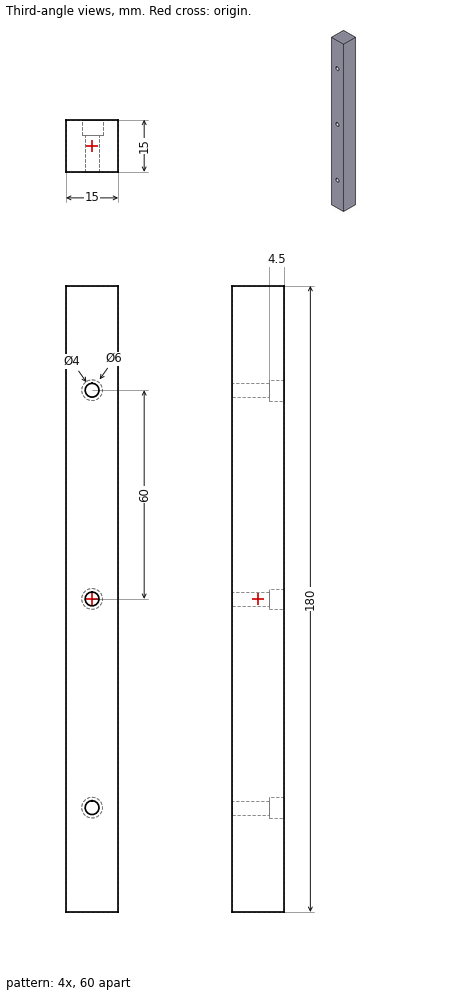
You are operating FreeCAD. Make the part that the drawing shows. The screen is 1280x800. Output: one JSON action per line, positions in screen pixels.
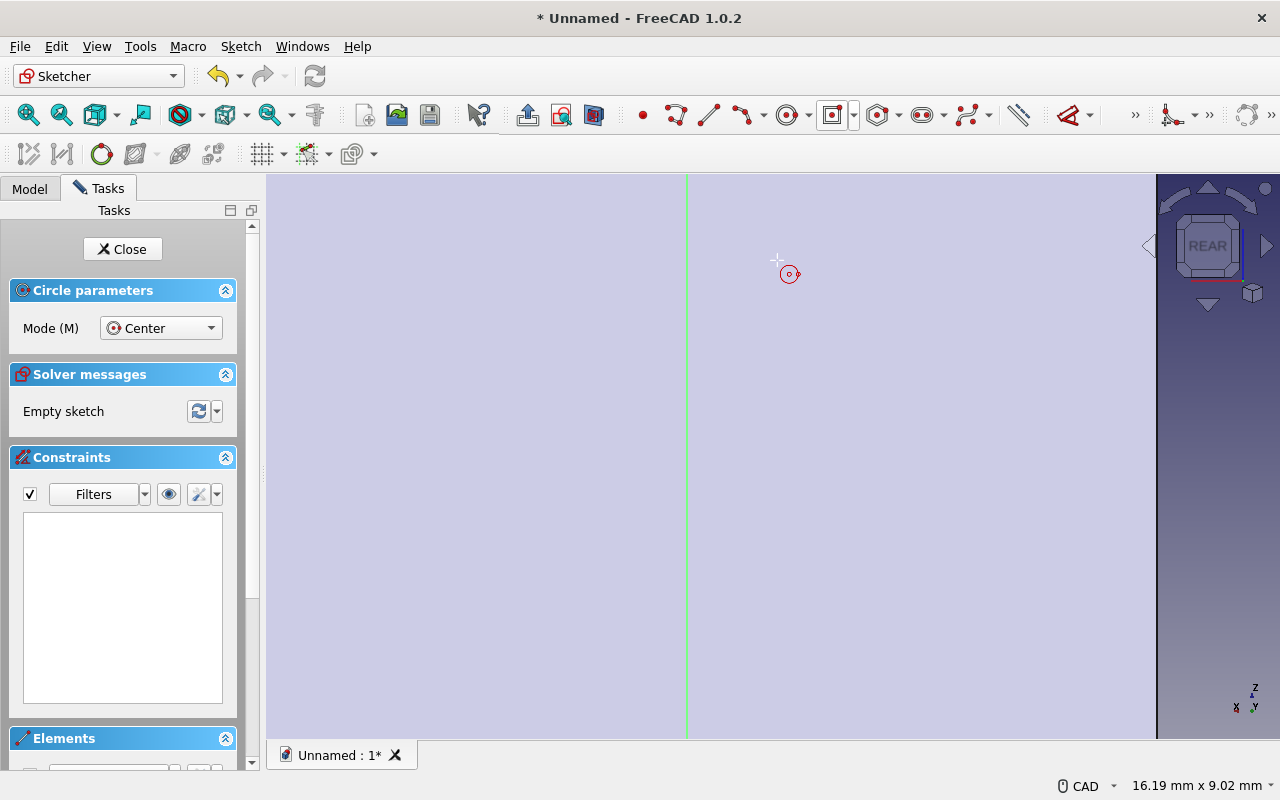
{"action": "left_click", "coordinate": [687, 447]}
{"action": "mouse_move", "coordinate": [820, 314]}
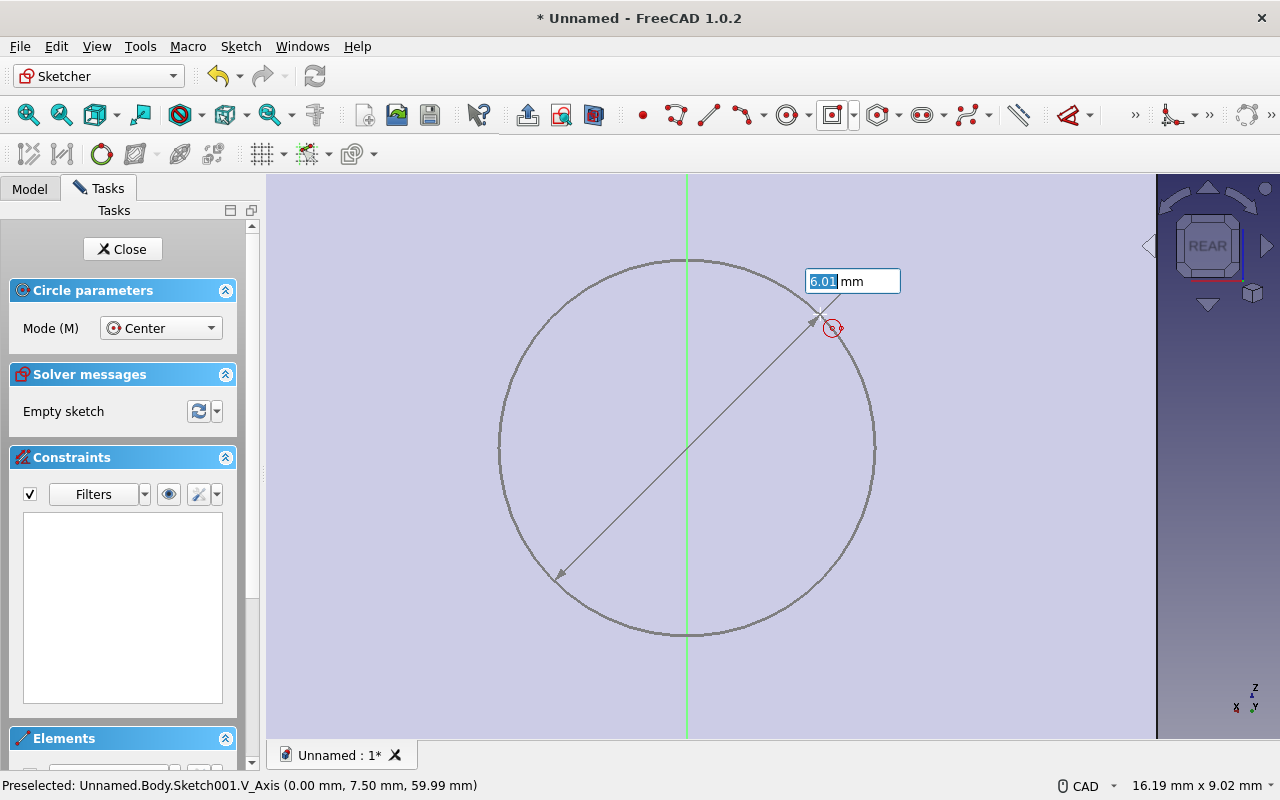
{"action": "type", "text": "6"}
{"action": "key", "text": "Return"}
{"action": "key", "text": "Escape"}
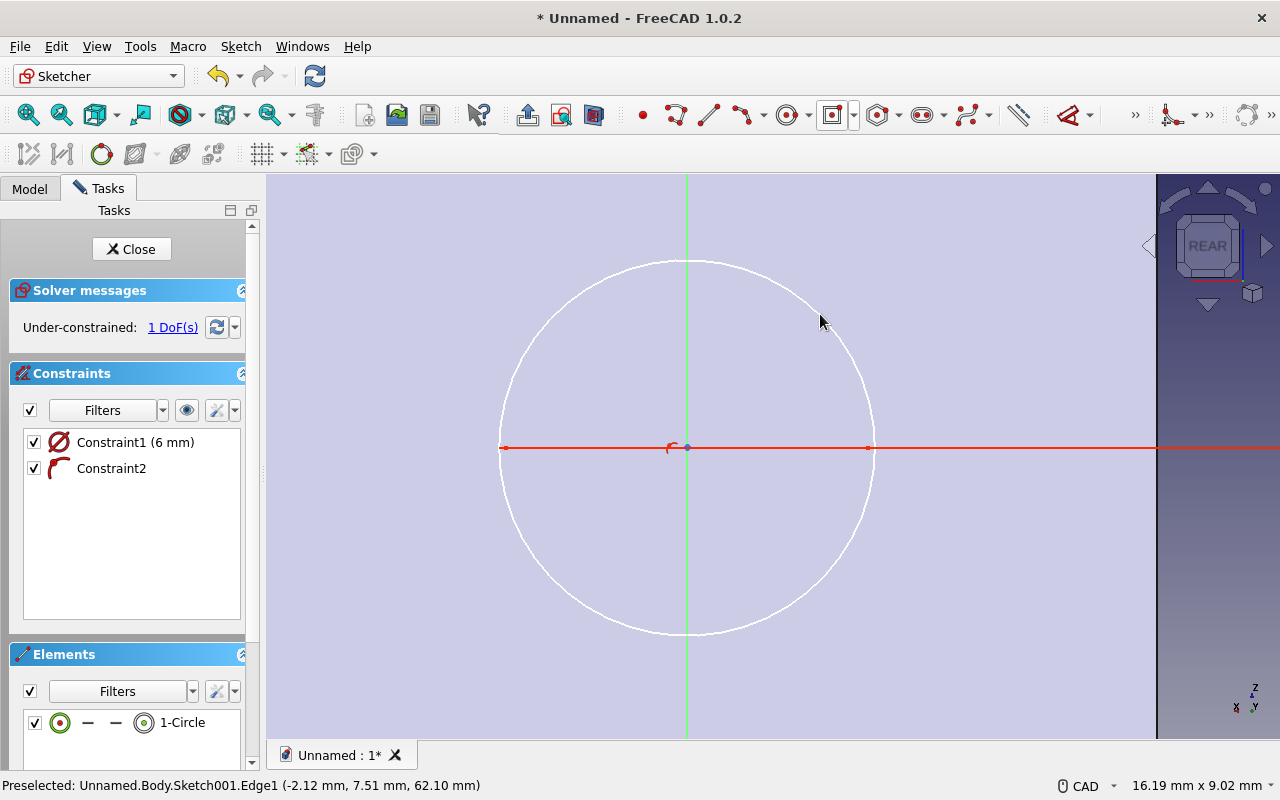
{"action": "left_click", "coordinate": [1068, 116]}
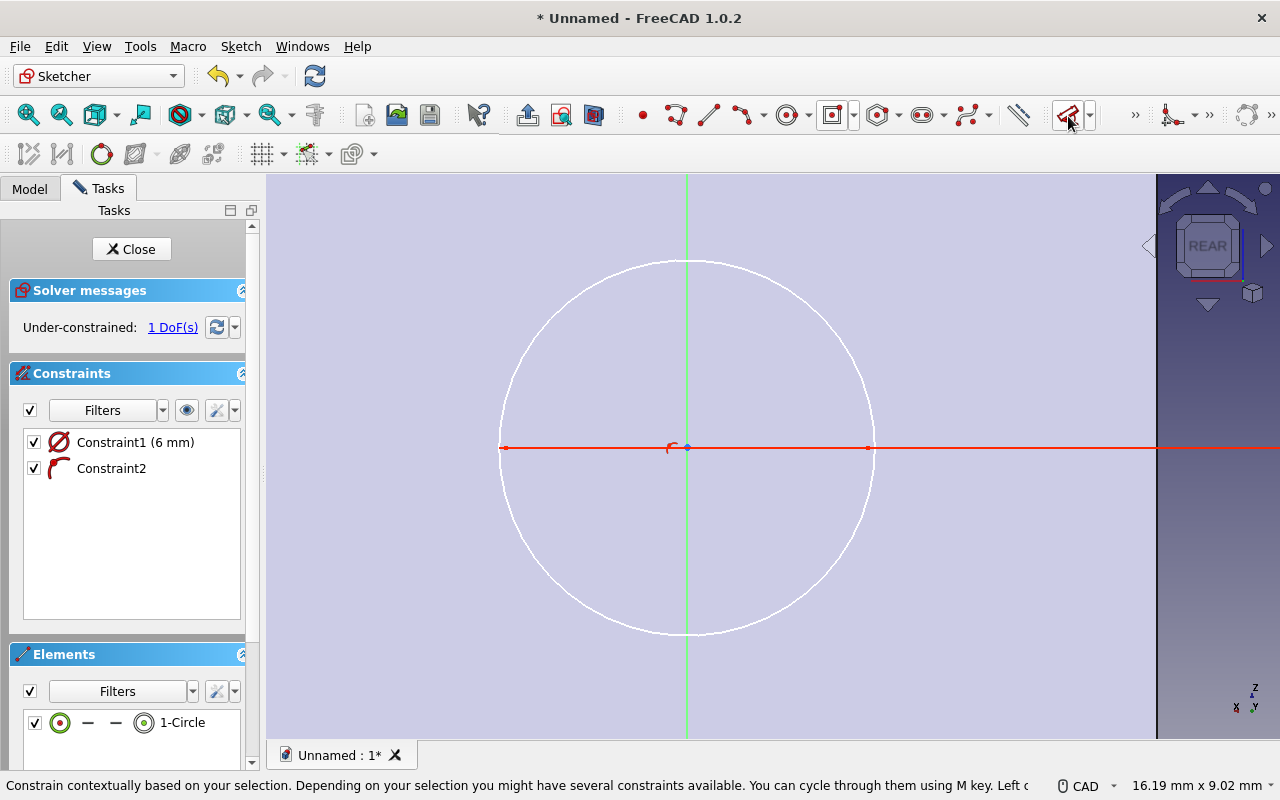
{"action": "left_click", "coordinate": [687, 448]}
{"action": "left_click", "coordinate": [721, 580]}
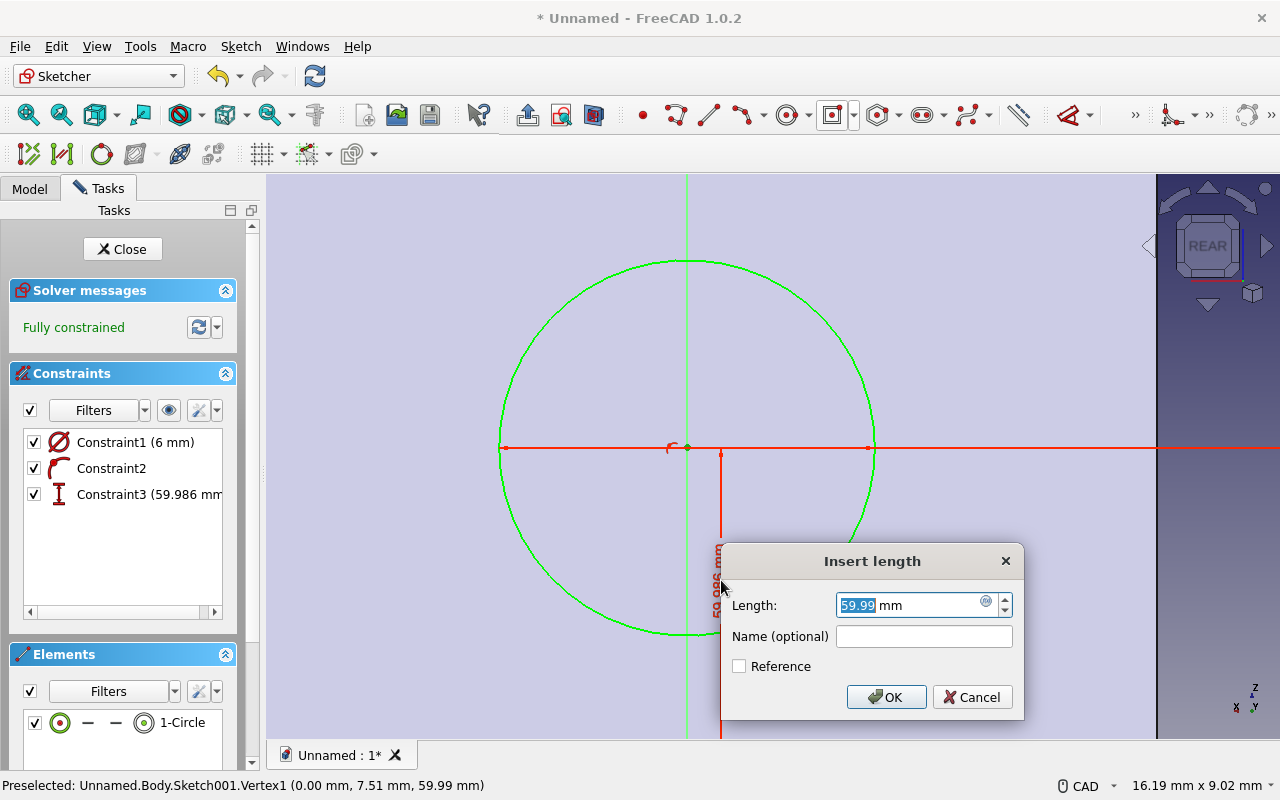
{"action": "type", "text": "60"}
{"action": "key", "text": "Return"}
{"action": "key", "text": "Escape"}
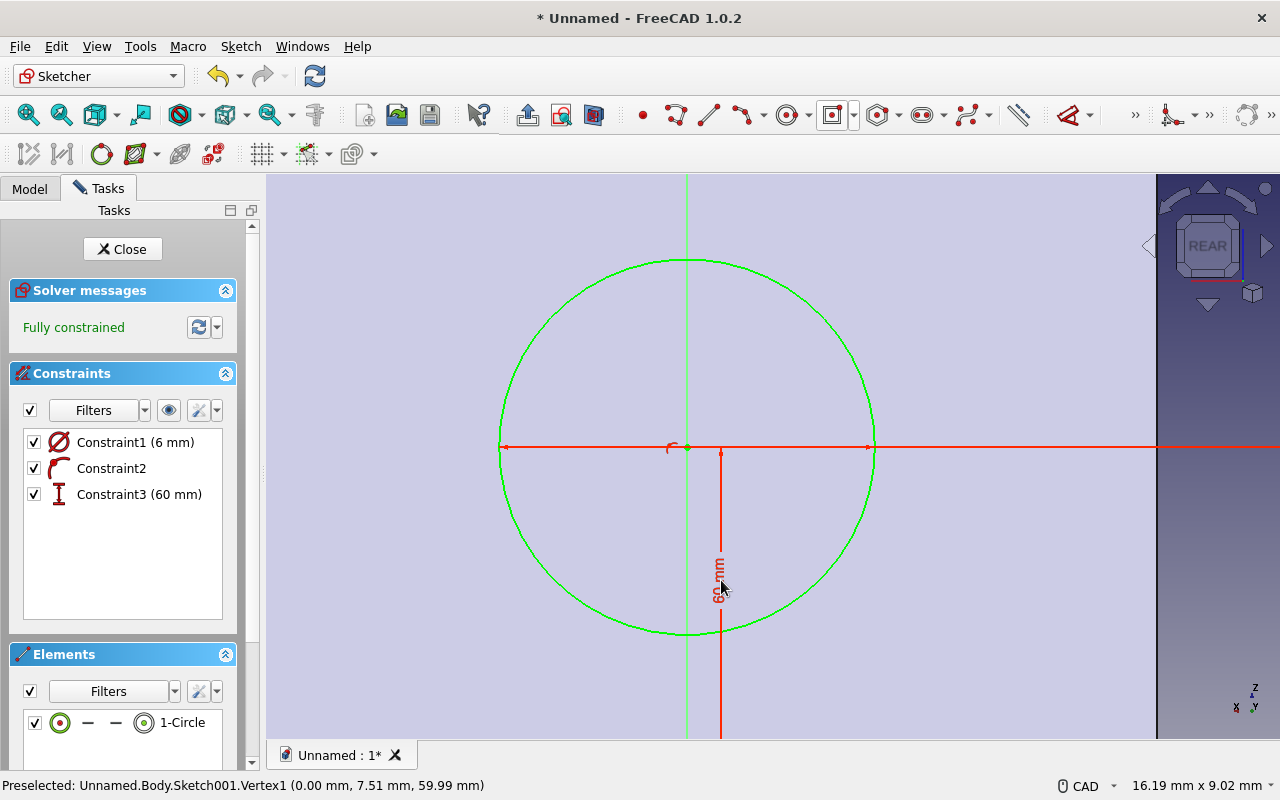
{"action": "left_click", "coordinate": [123, 249]}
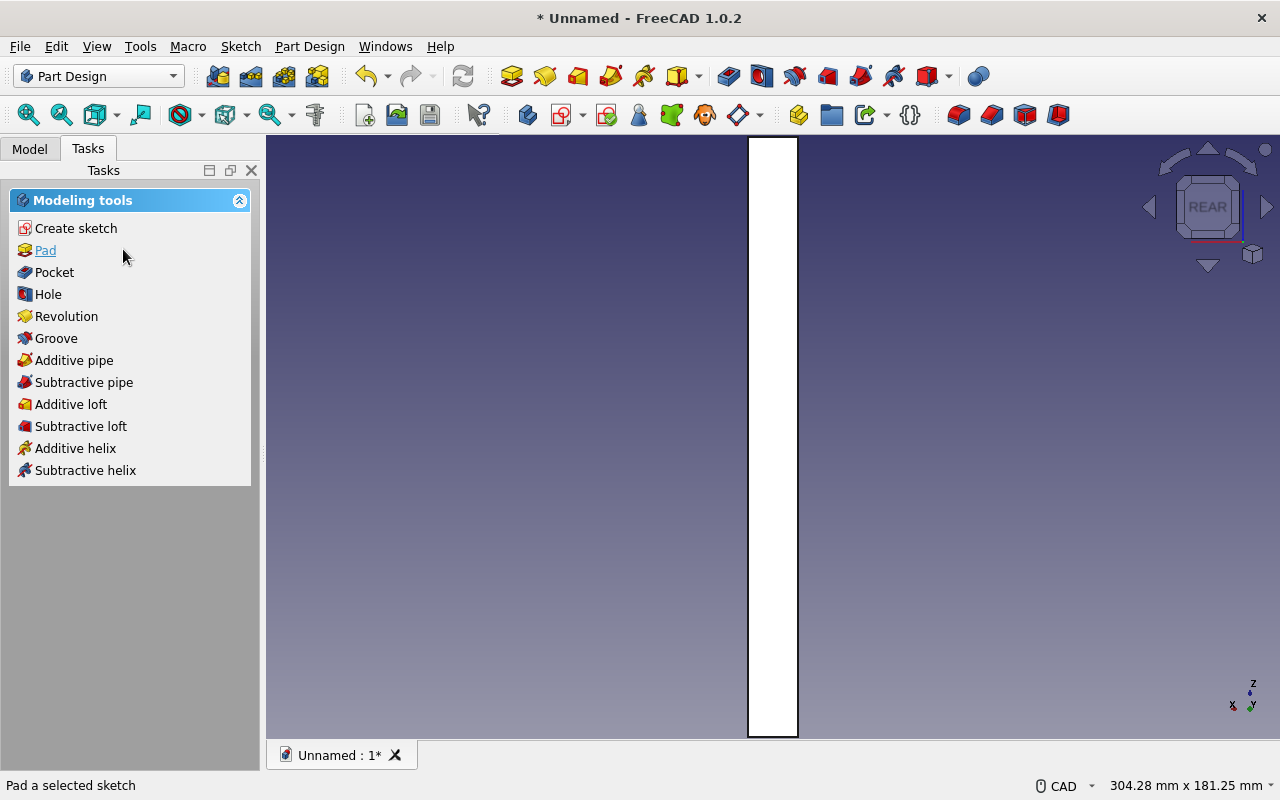
{"action": "left_click", "coordinate": [729, 76]}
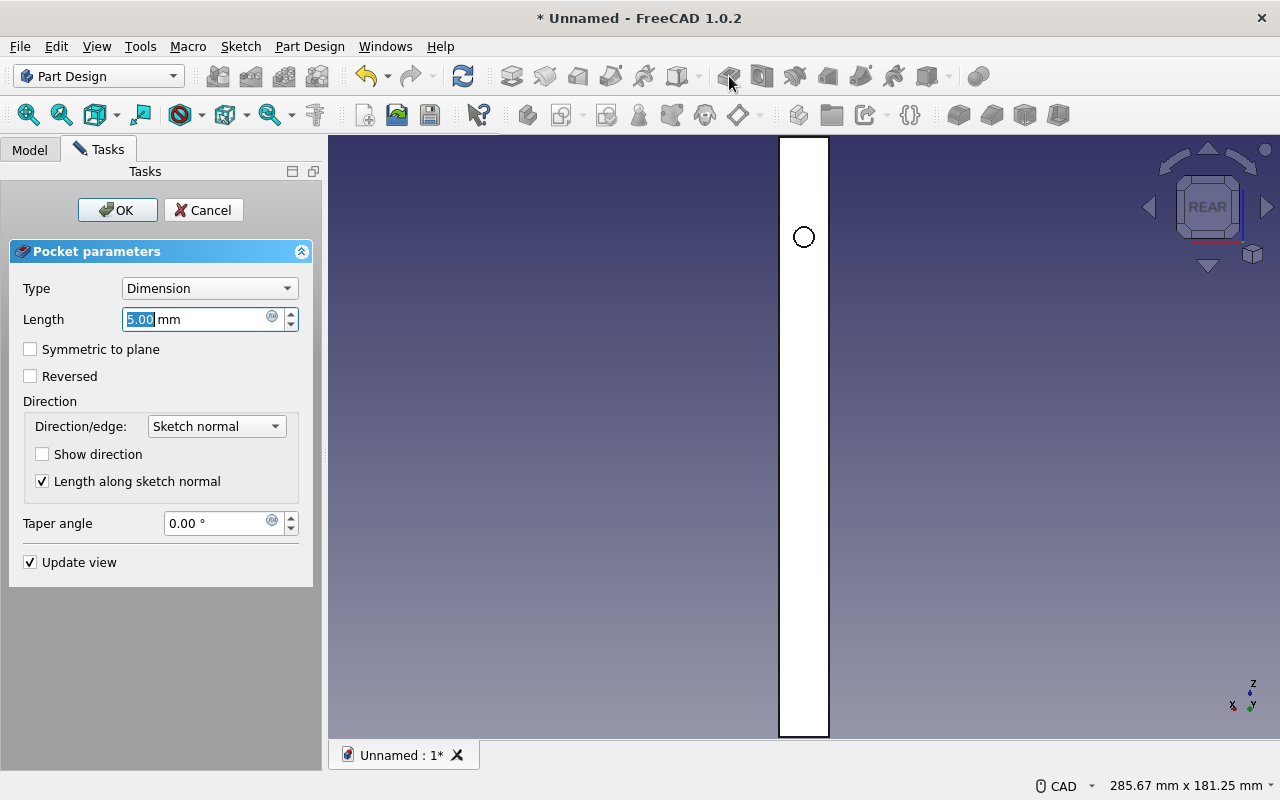
{"action": "type", "text": "4.5"}
{"action": "key", "text": "Tab"}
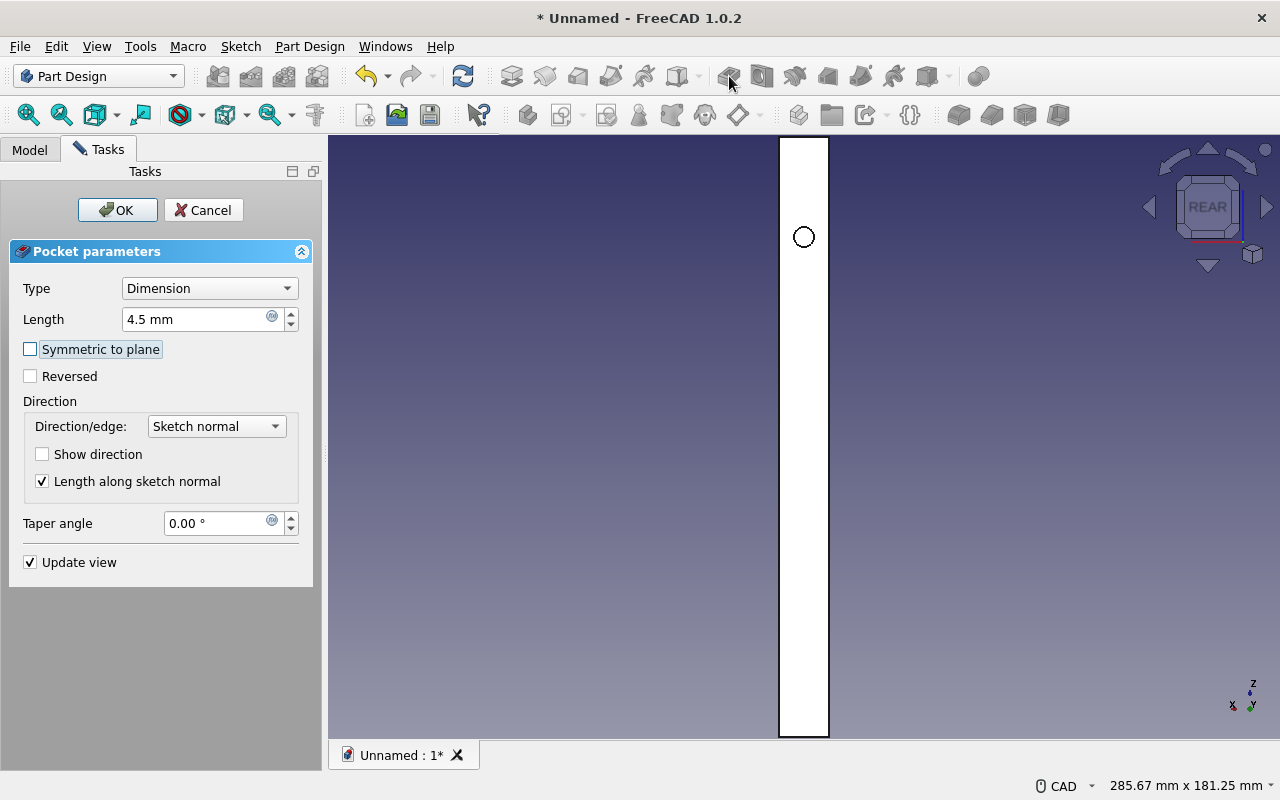
{"action": "left_click", "coordinate": [118, 210]}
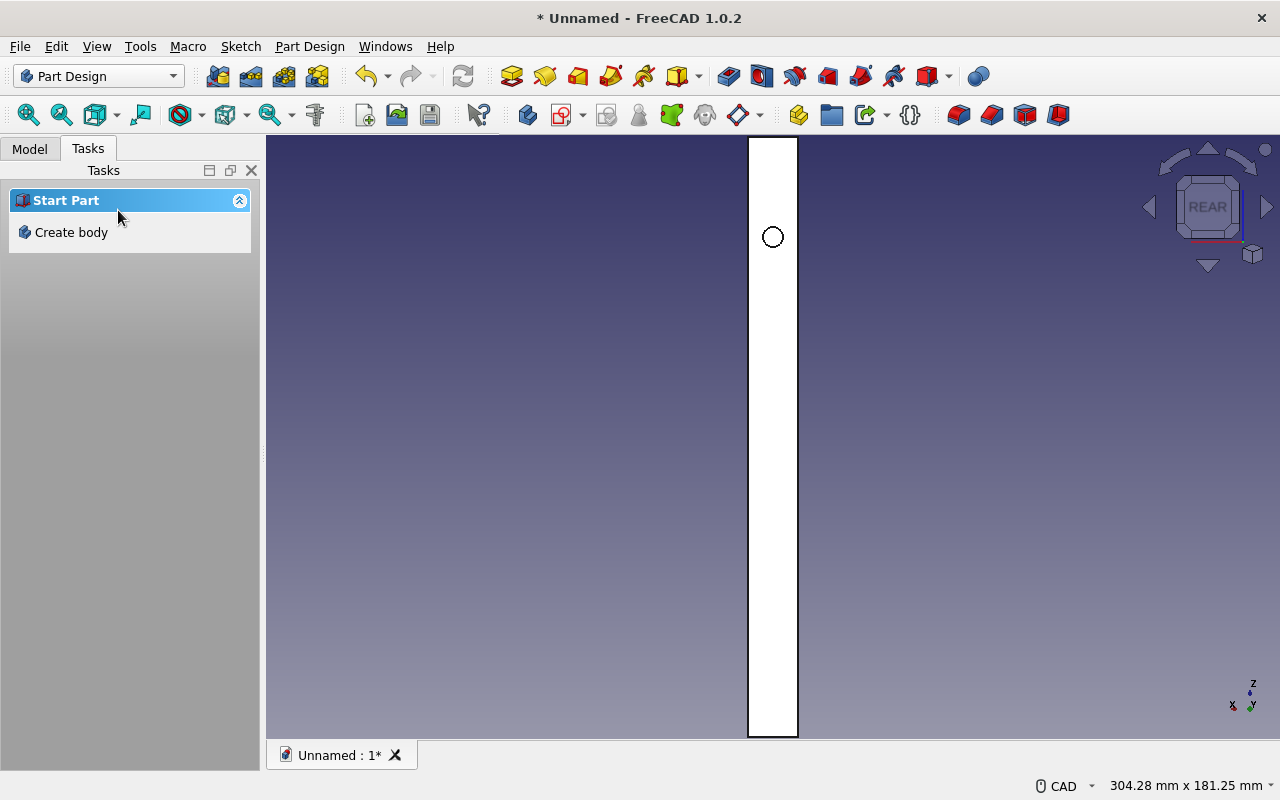
{"action": "left_click", "coordinate": [773, 179]}